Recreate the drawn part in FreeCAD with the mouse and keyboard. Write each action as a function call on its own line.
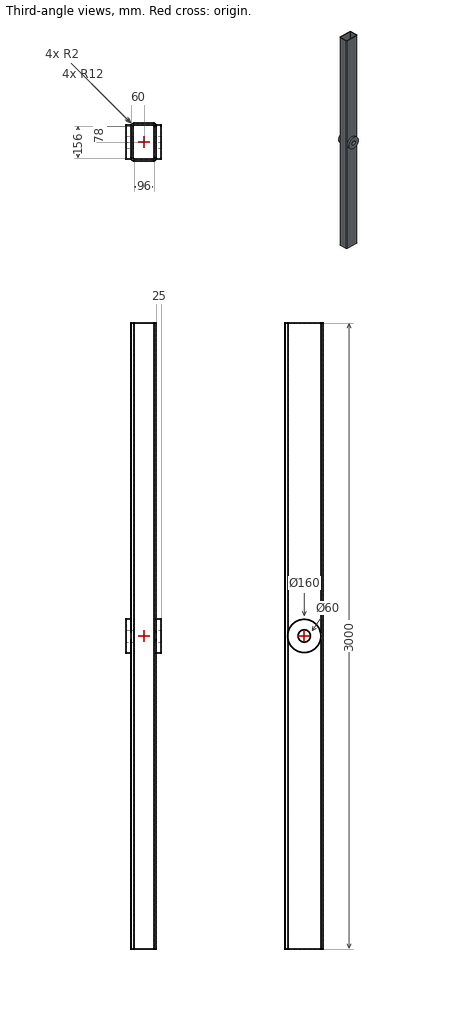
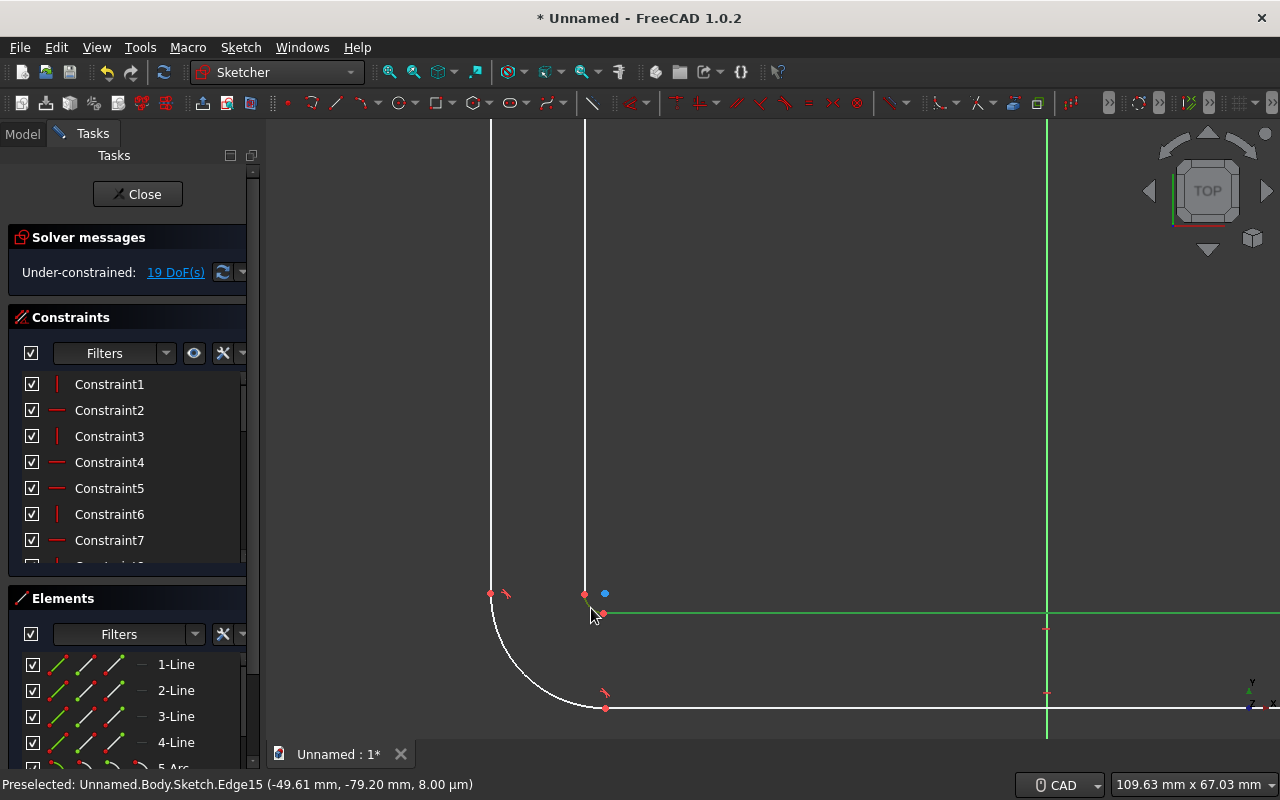
click(786, 104)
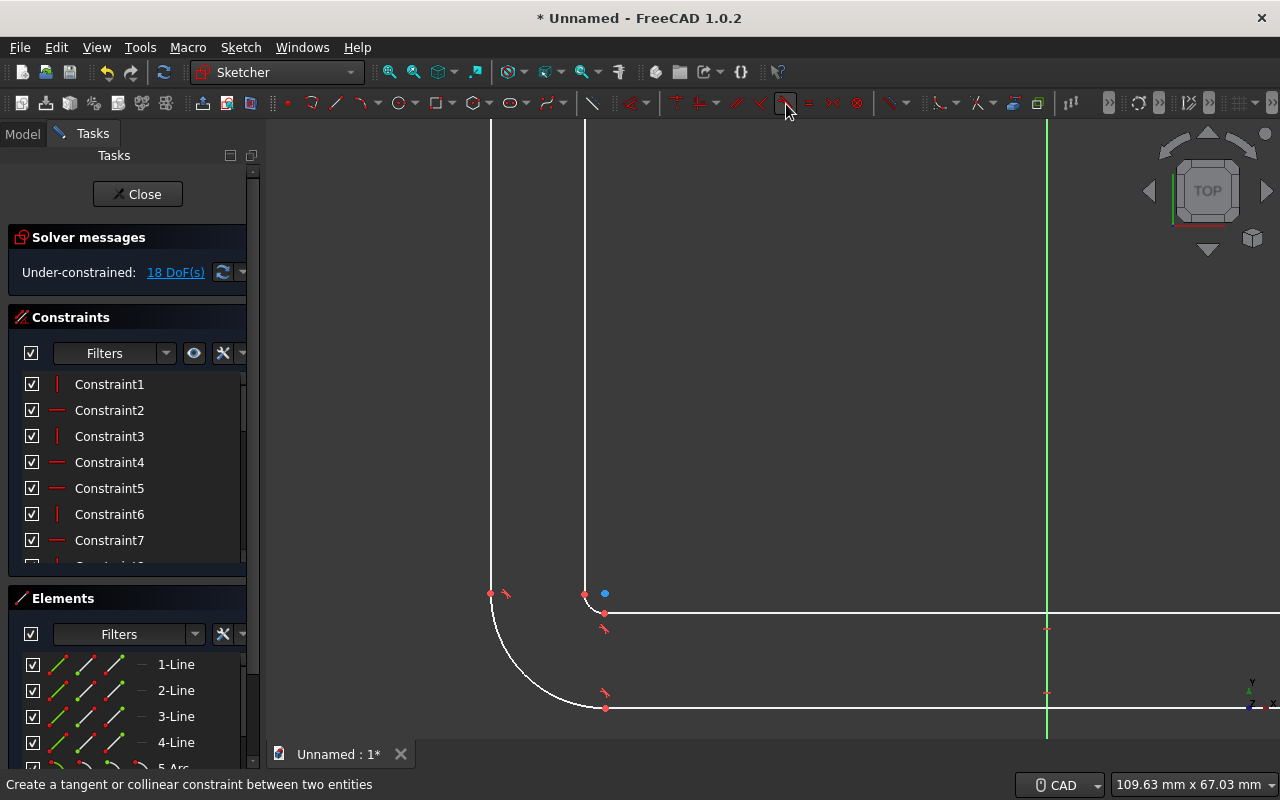
scroll(592, 611, down, 7)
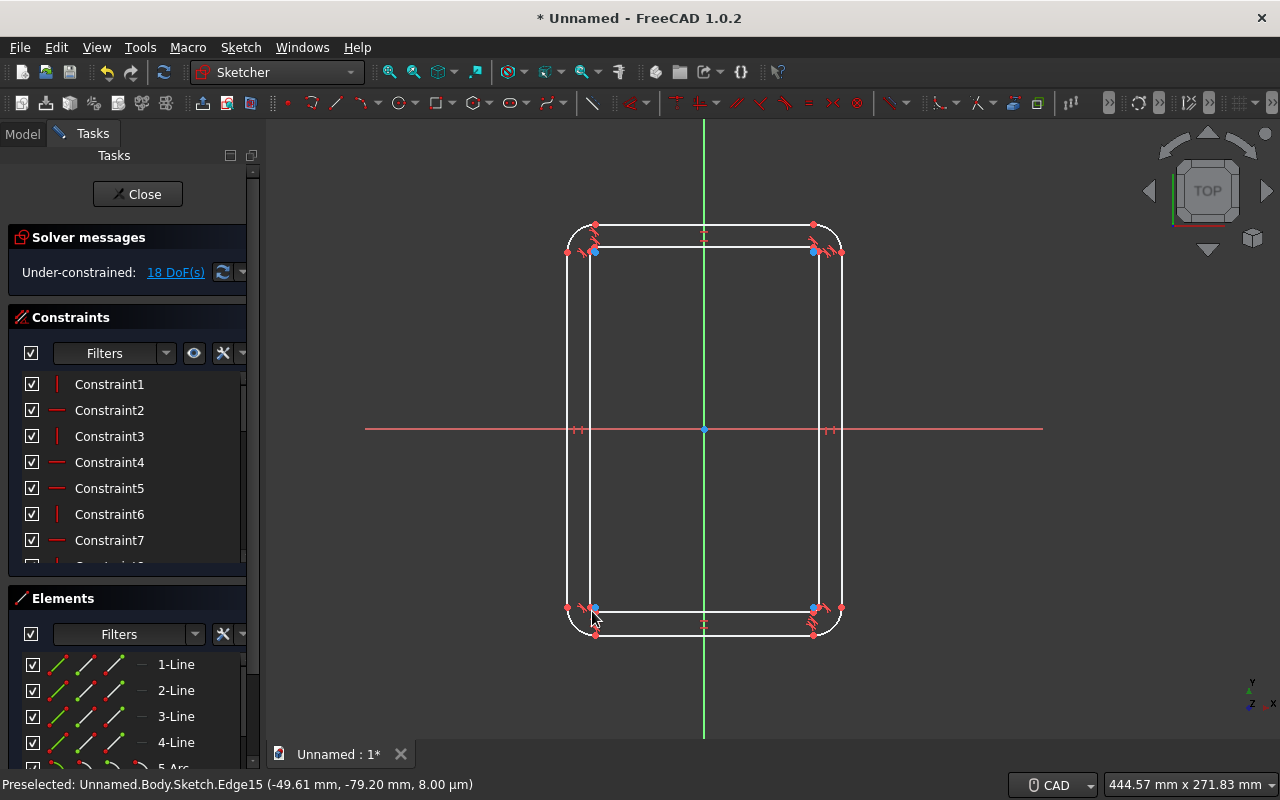
click(590, 501)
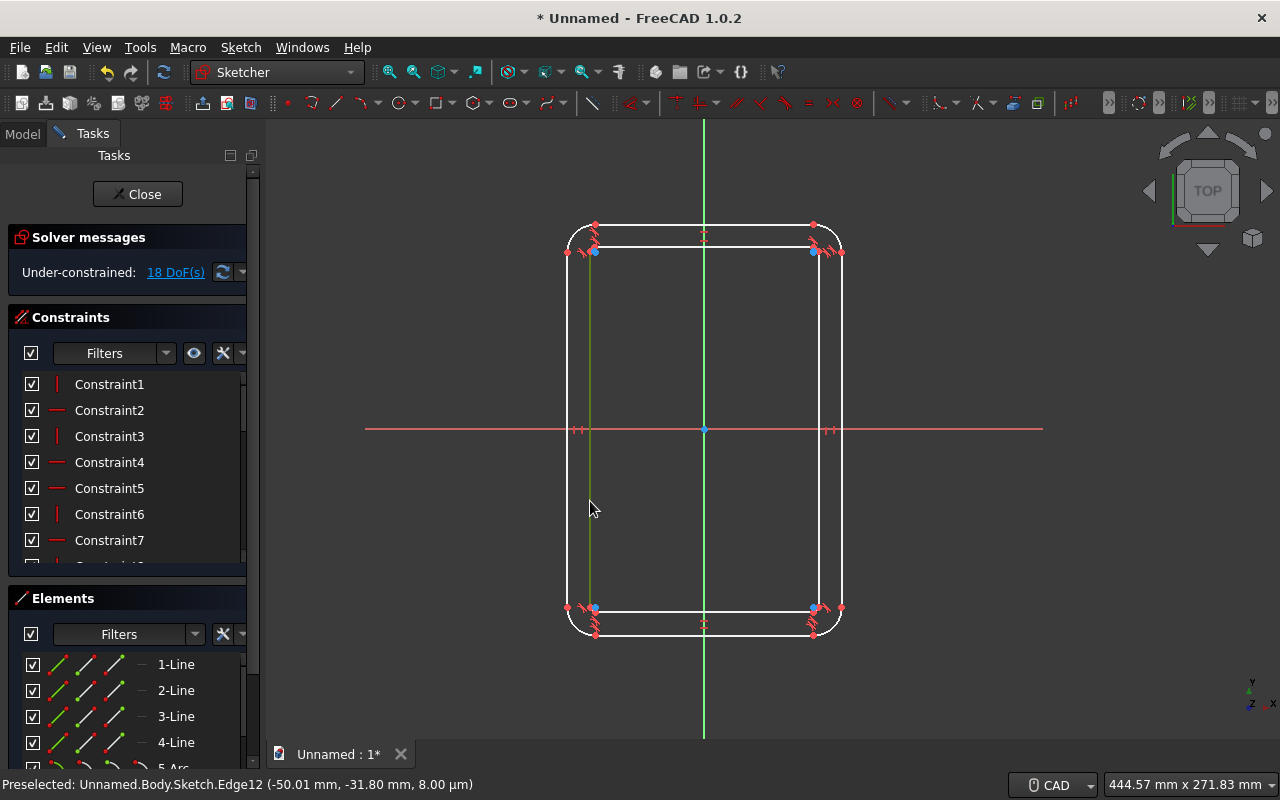
scroll(592, 611, up, 7)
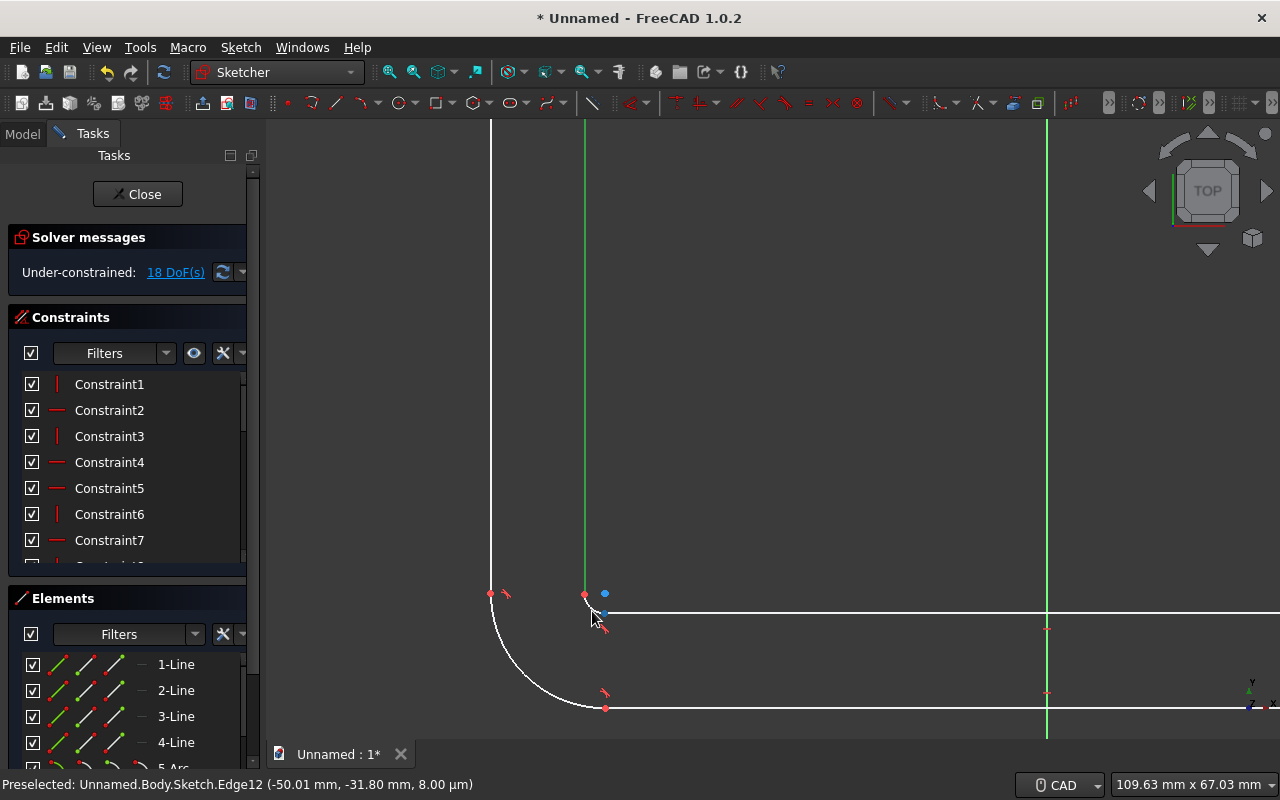
click(591, 608)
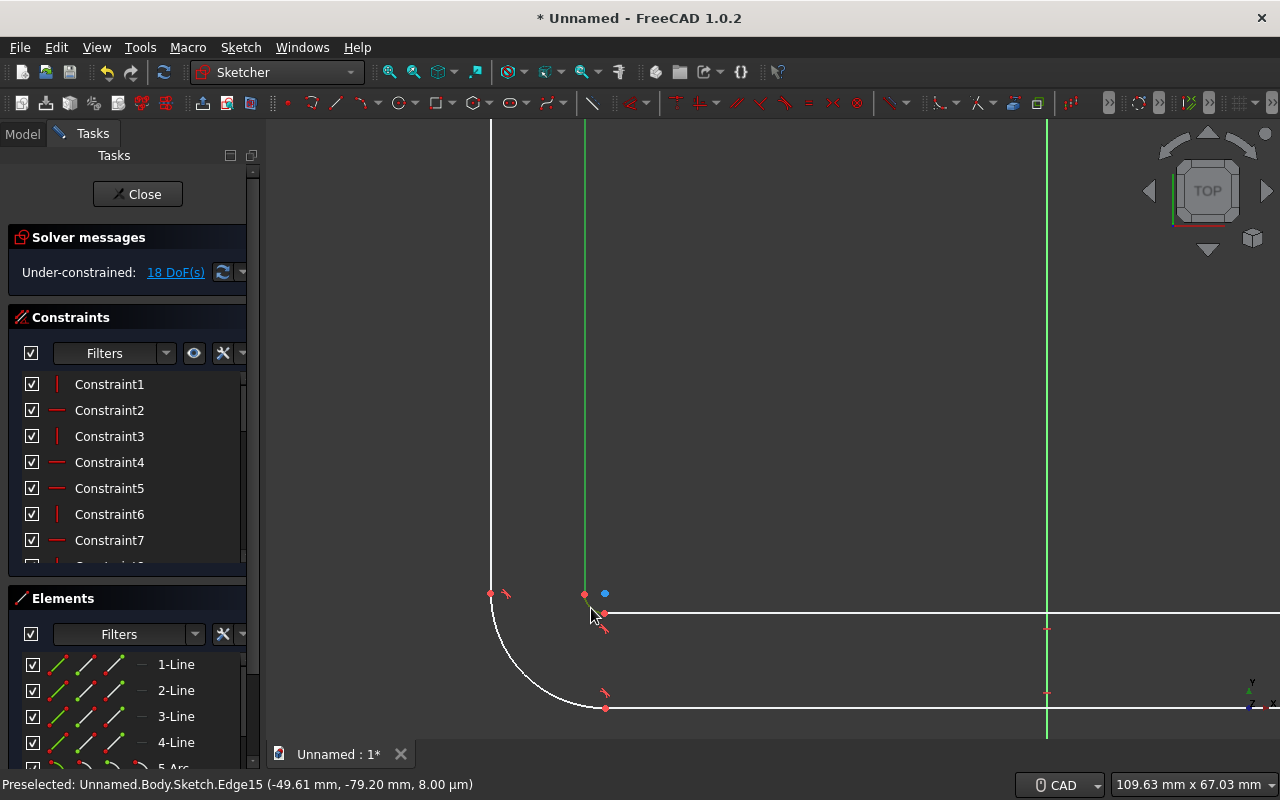
click(786, 104)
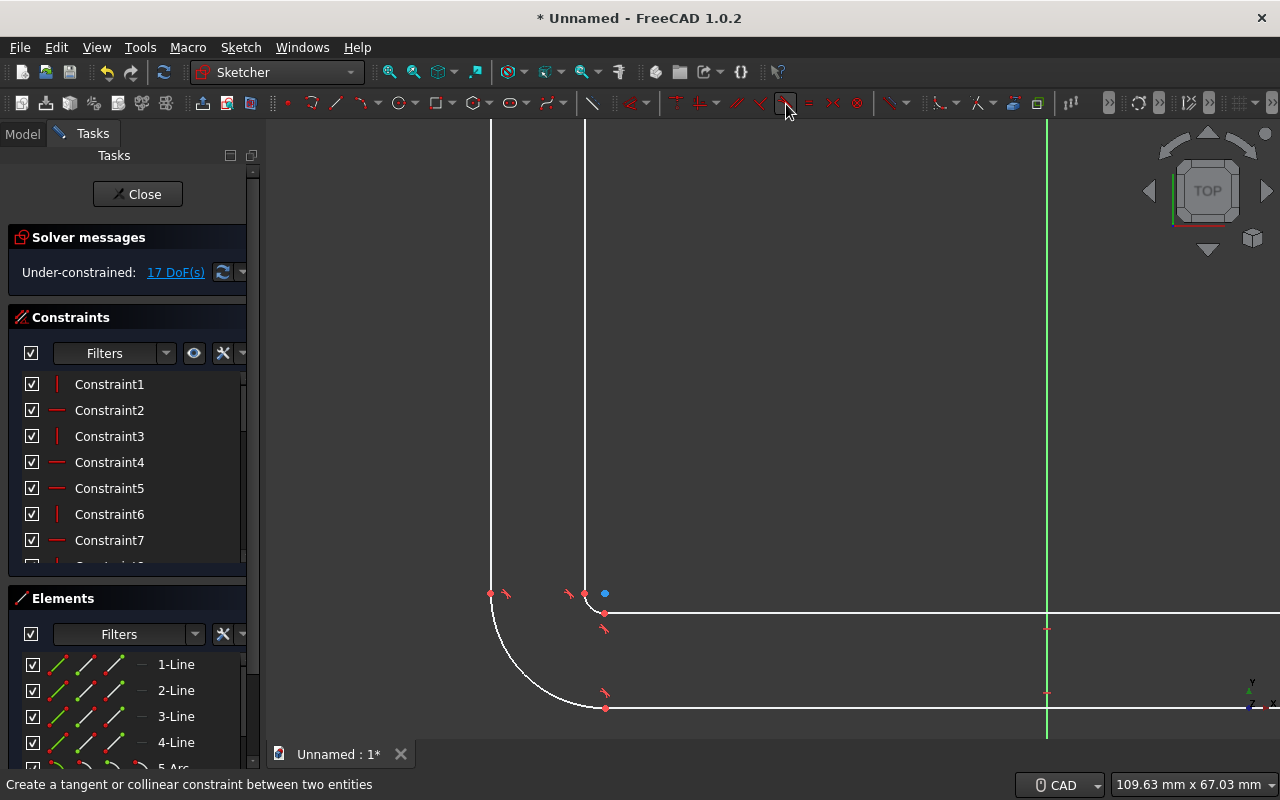
scroll(592, 611, down, 7)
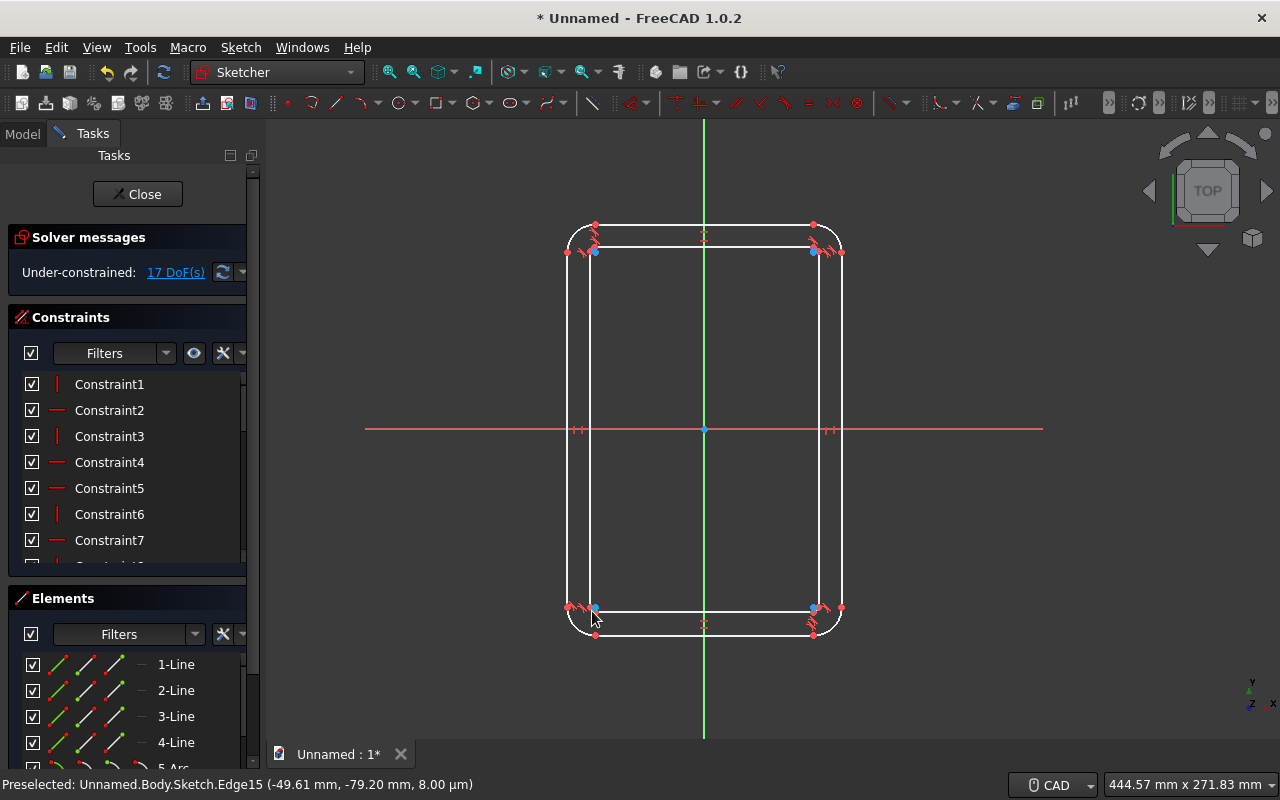
click(590, 501)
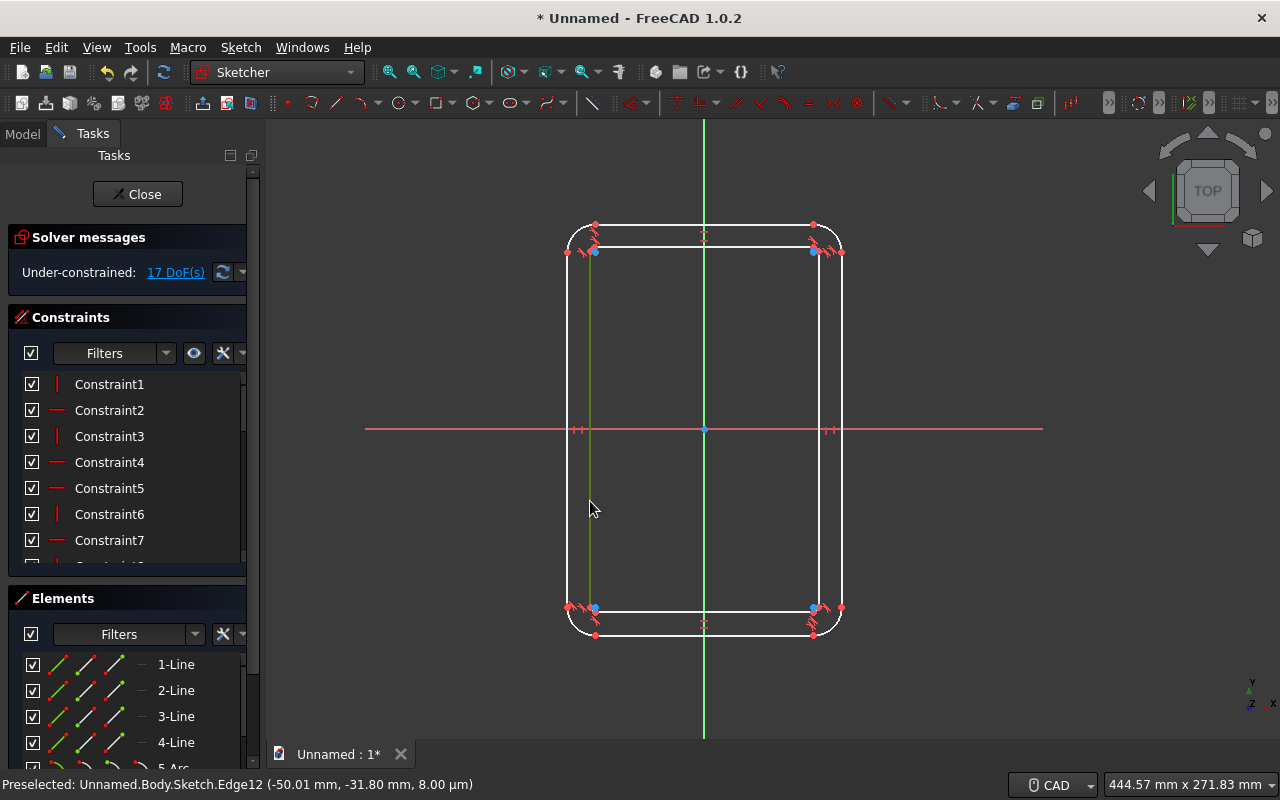
scroll(592, 248, up, 7)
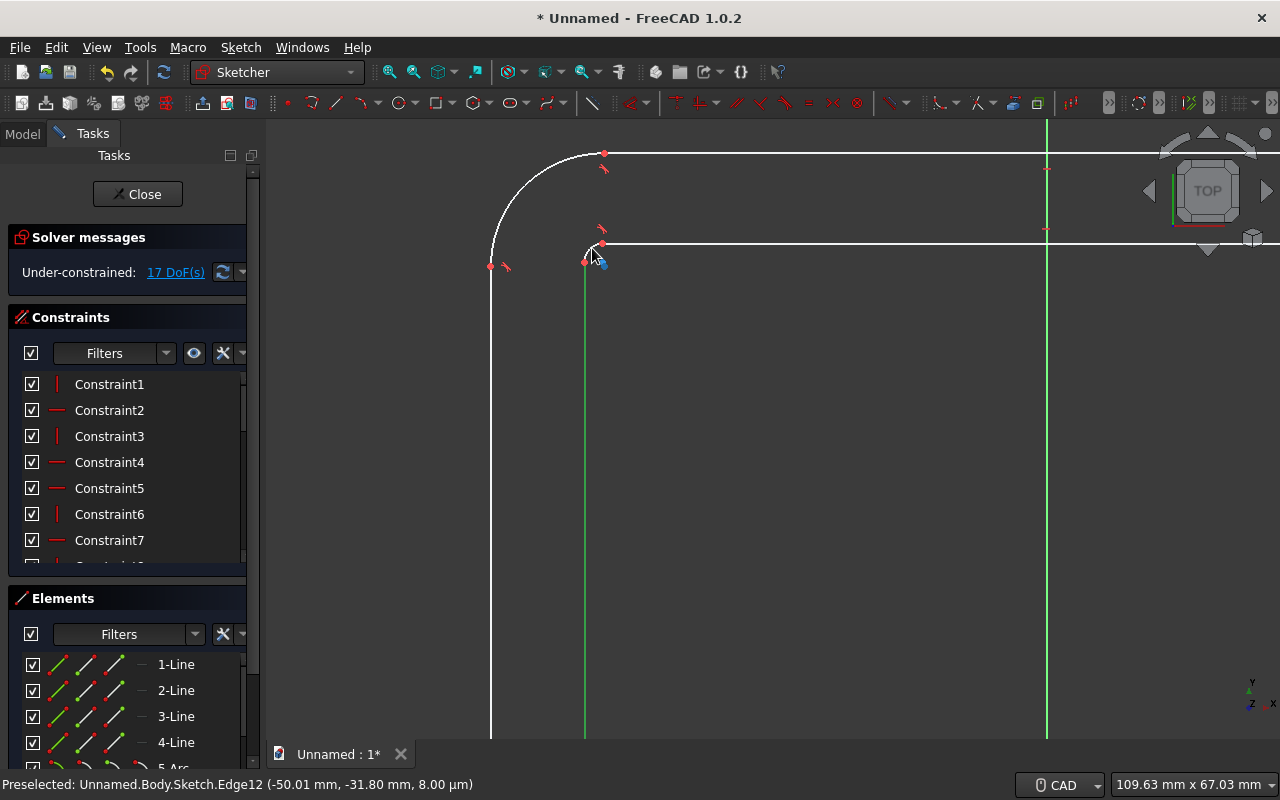
click(590, 249)